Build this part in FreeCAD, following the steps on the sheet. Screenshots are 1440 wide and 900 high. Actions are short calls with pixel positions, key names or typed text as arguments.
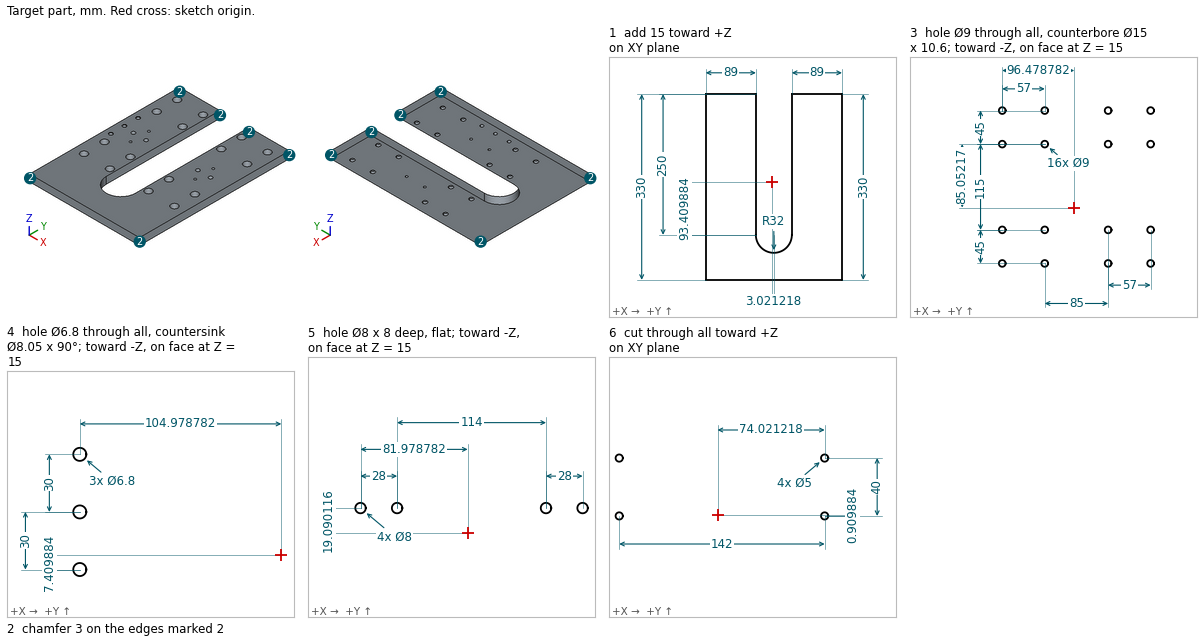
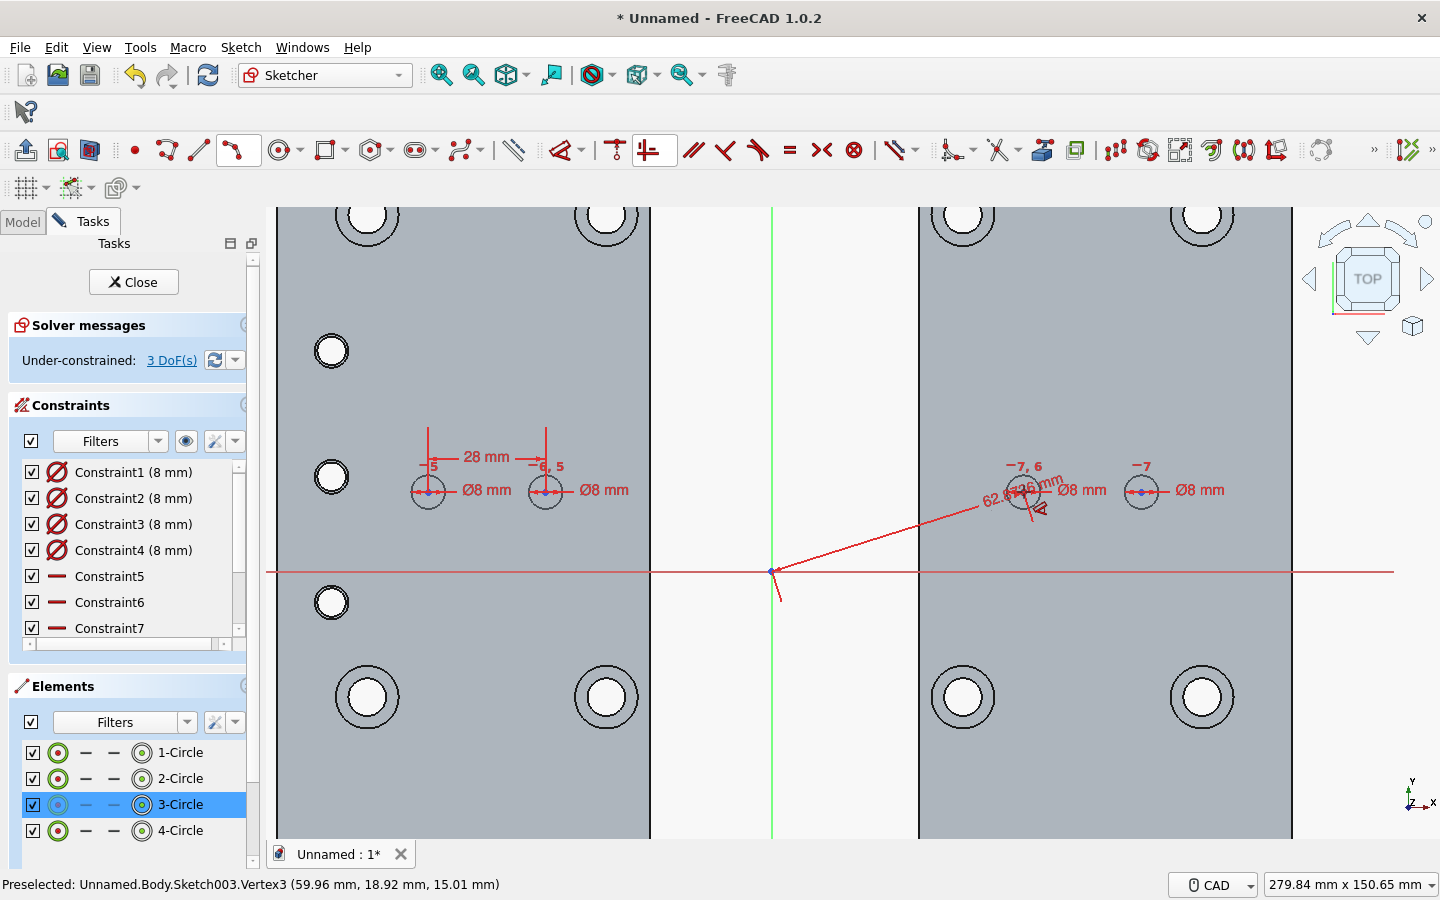
click(1142, 492)
click(1083, 458)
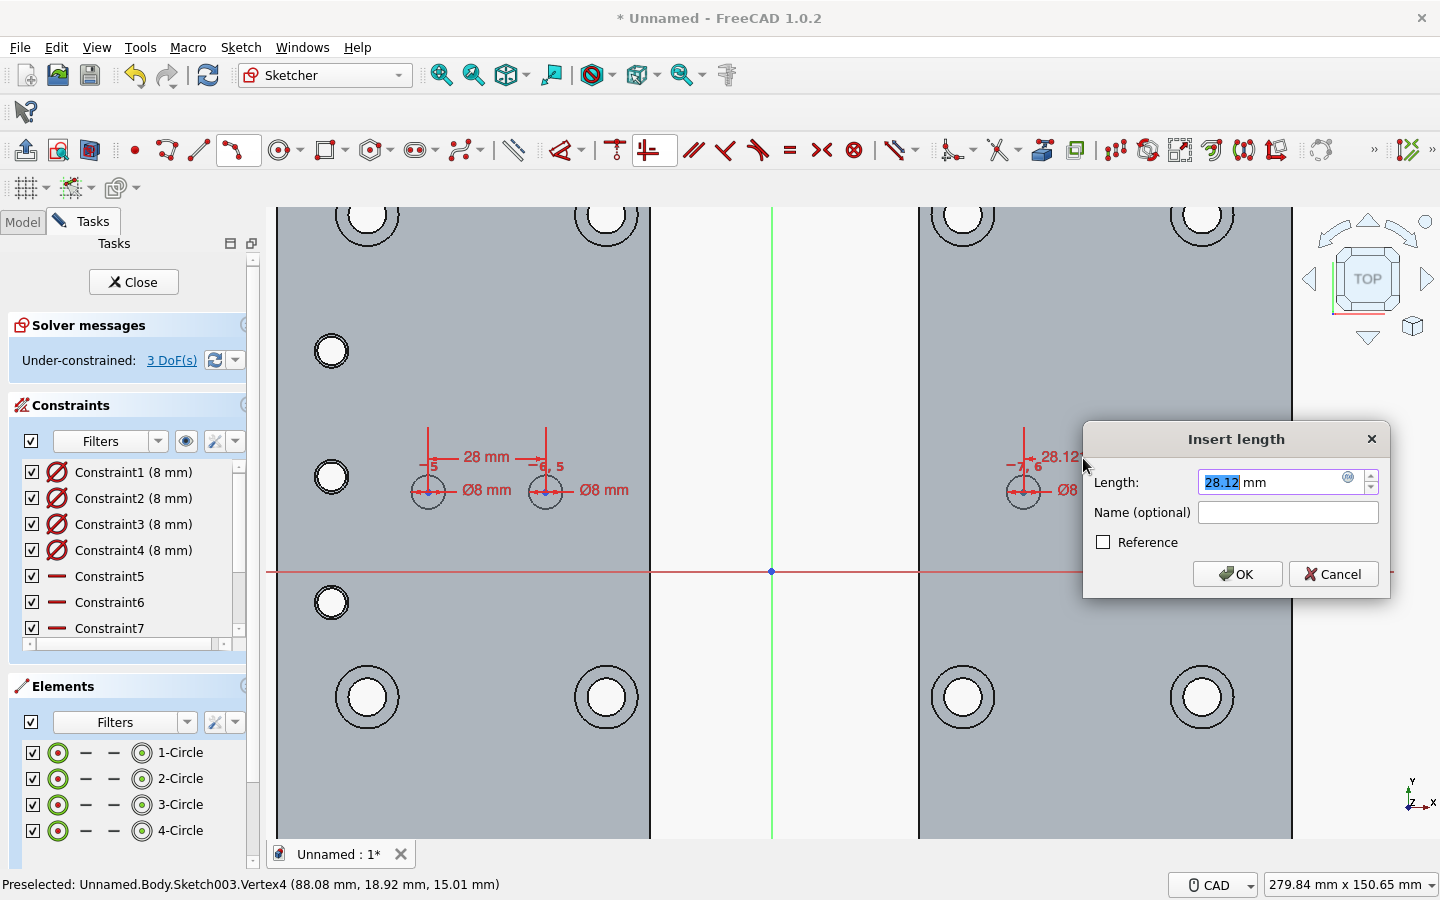
text(28)
key(Return)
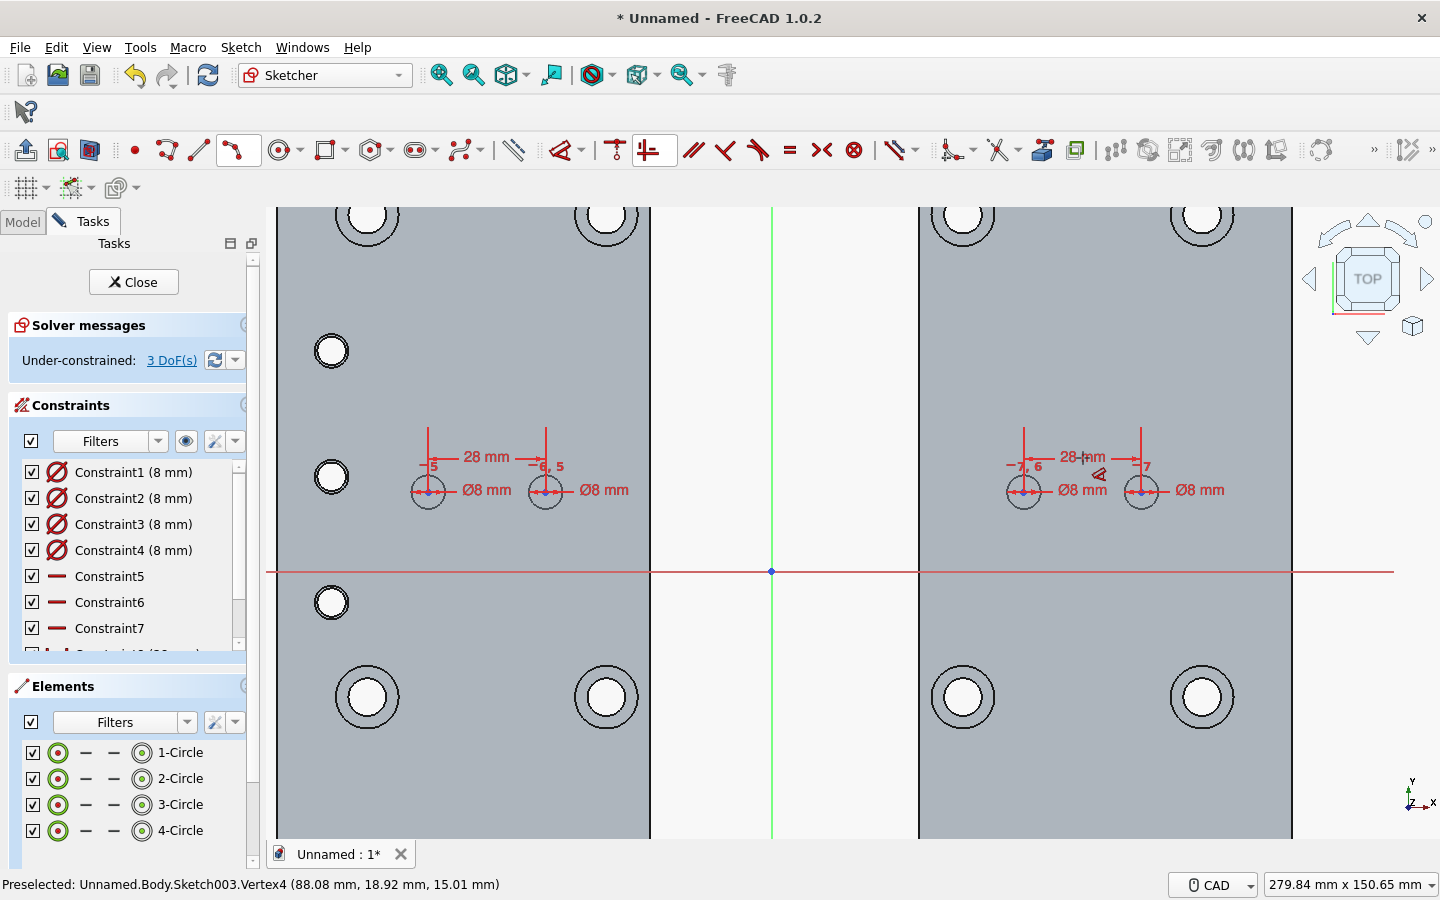
click(546, 492)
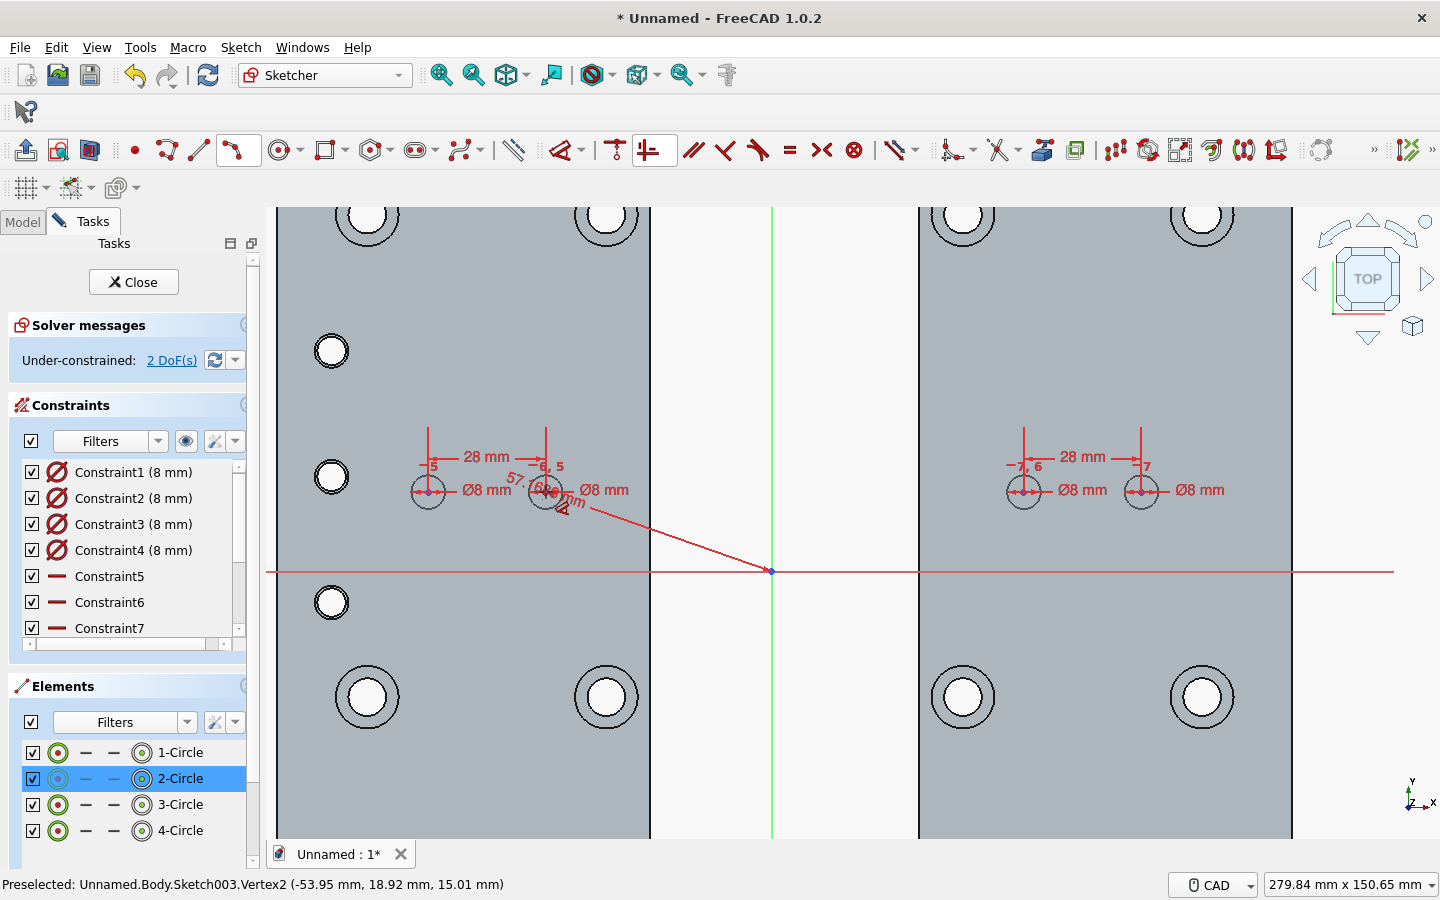
click(1024, 492)
click(675, 458)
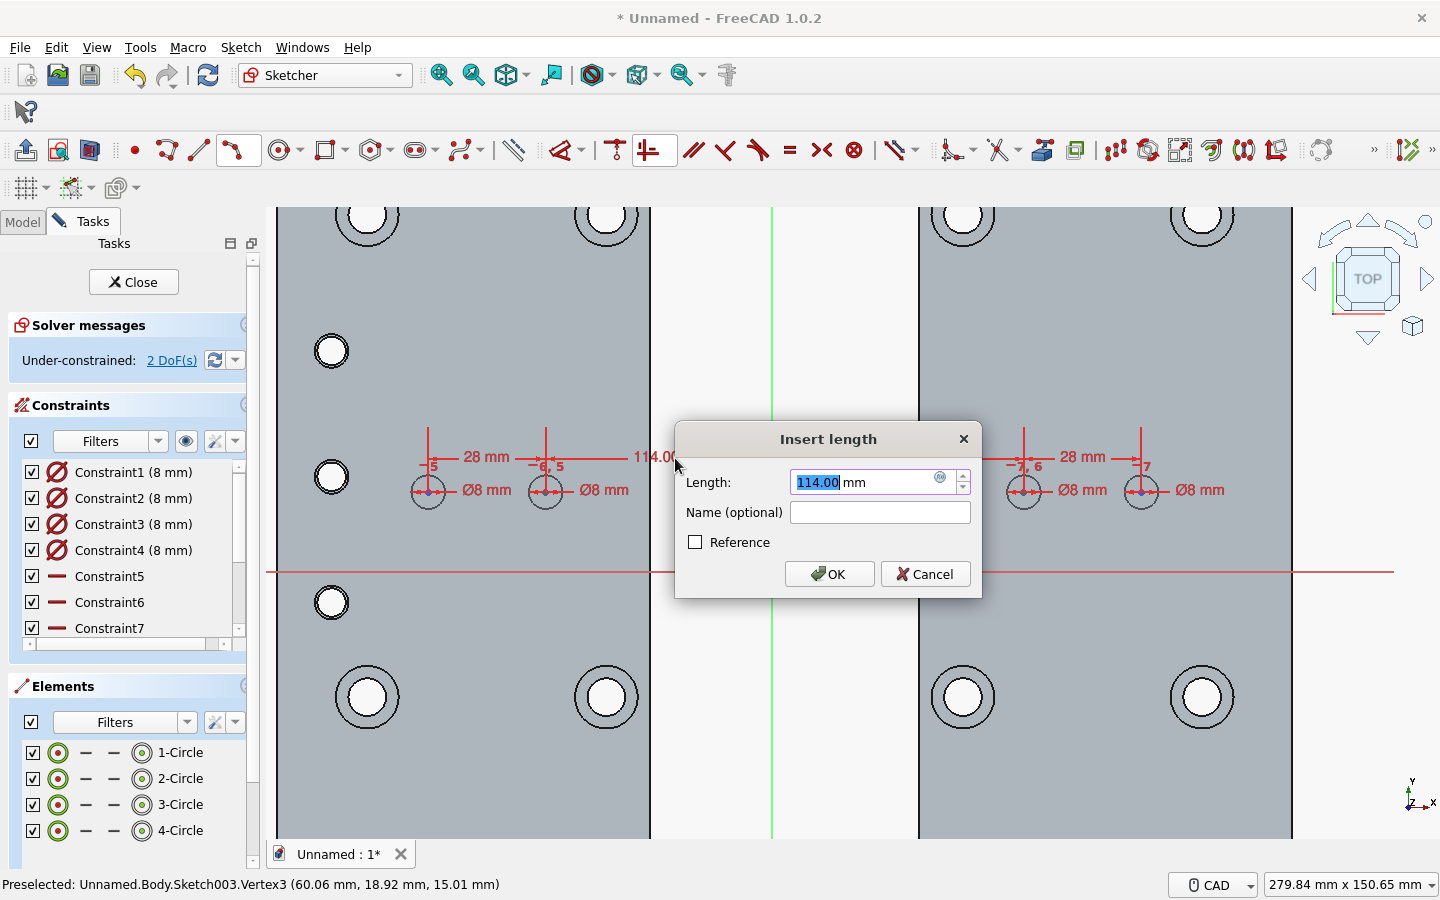
text(114)
key(Return)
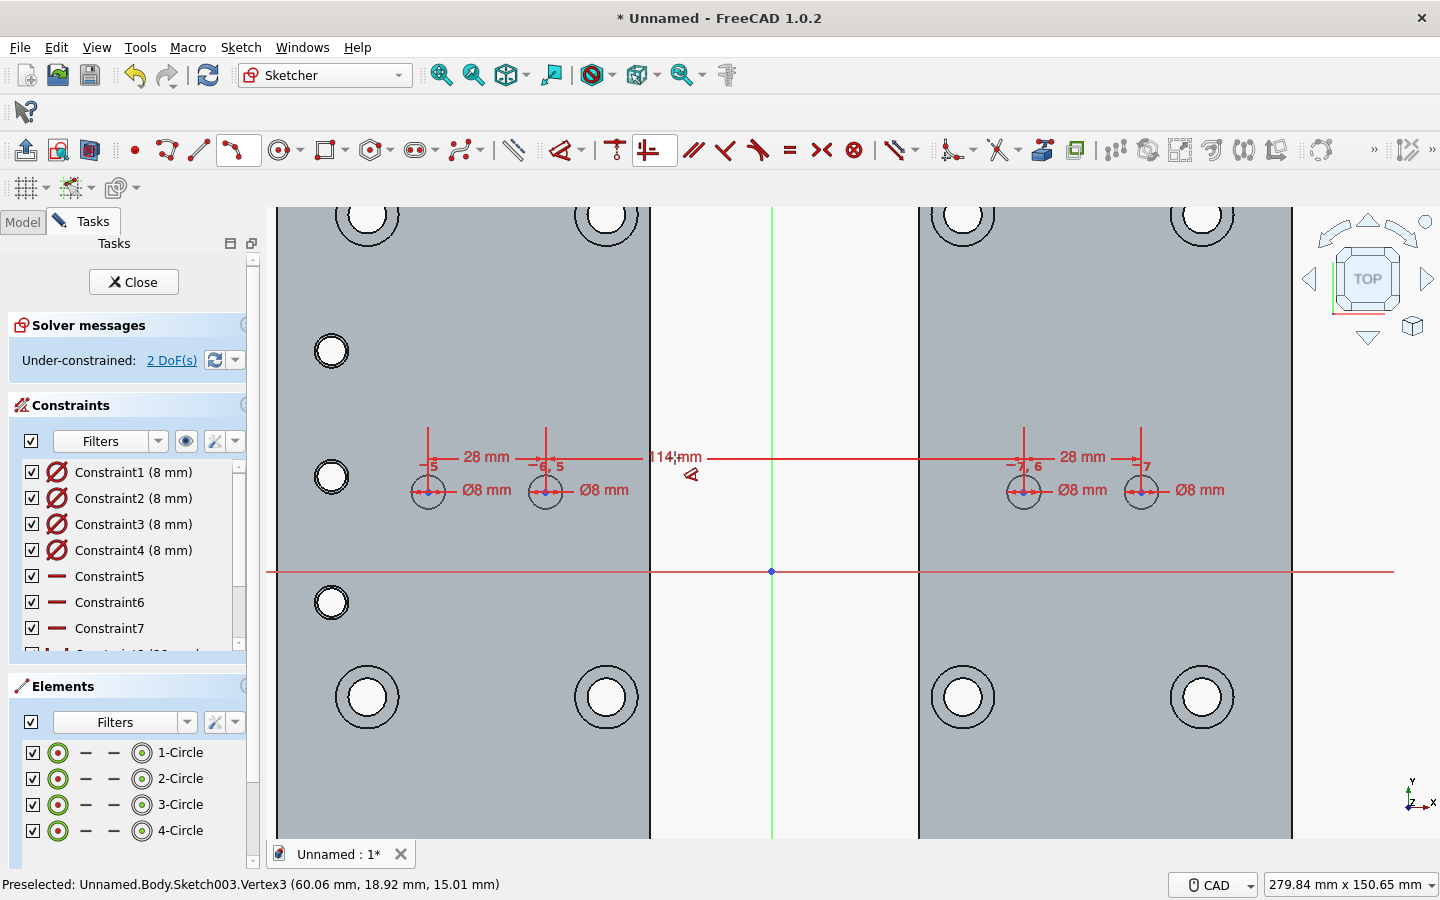
click(428, 492)
click(600, 606)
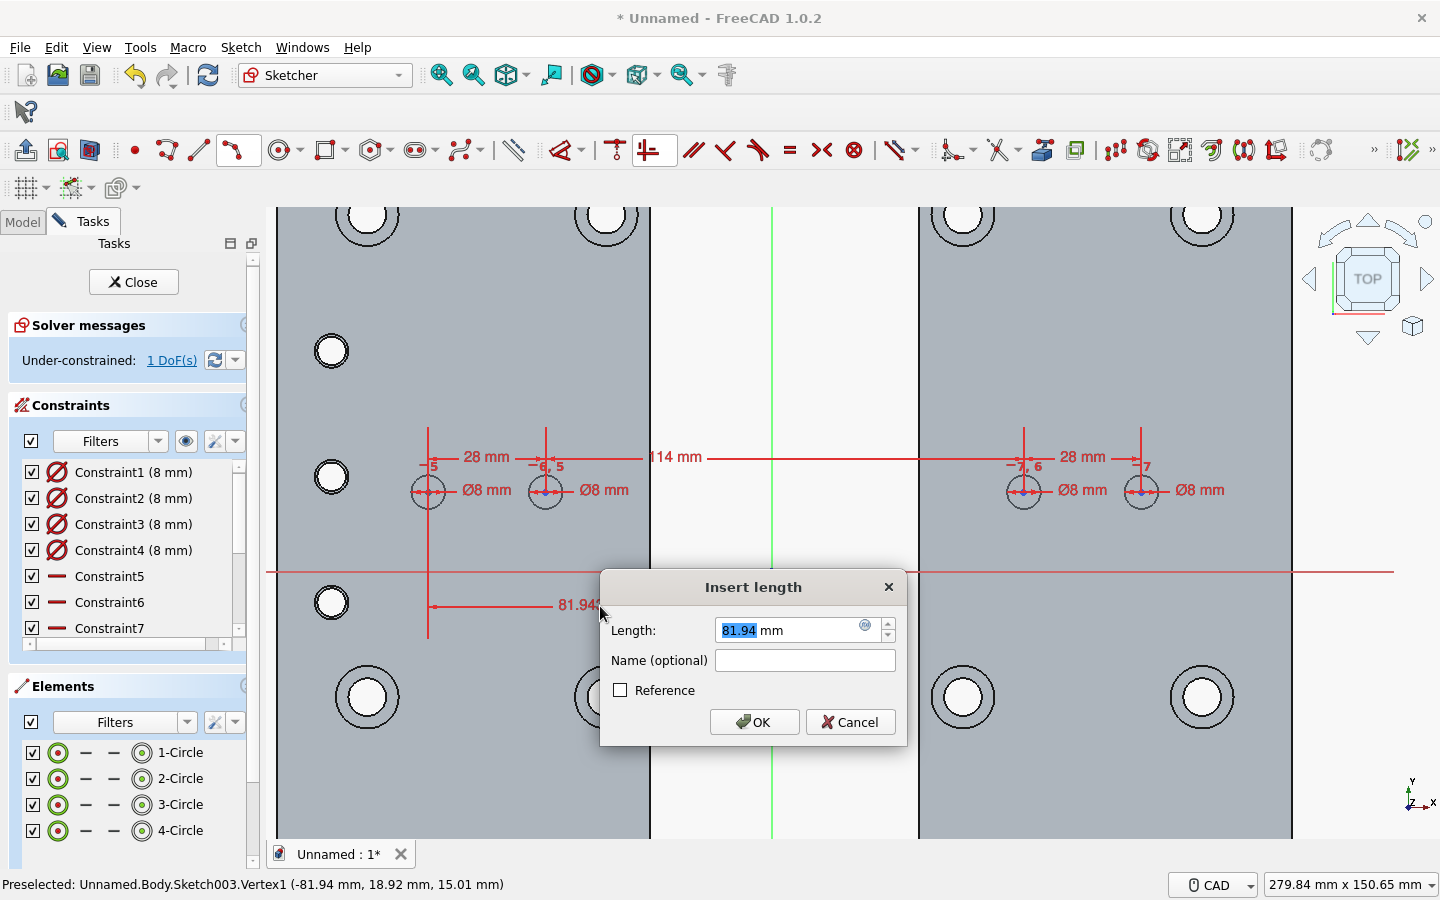
text(81.978782)
key(Return)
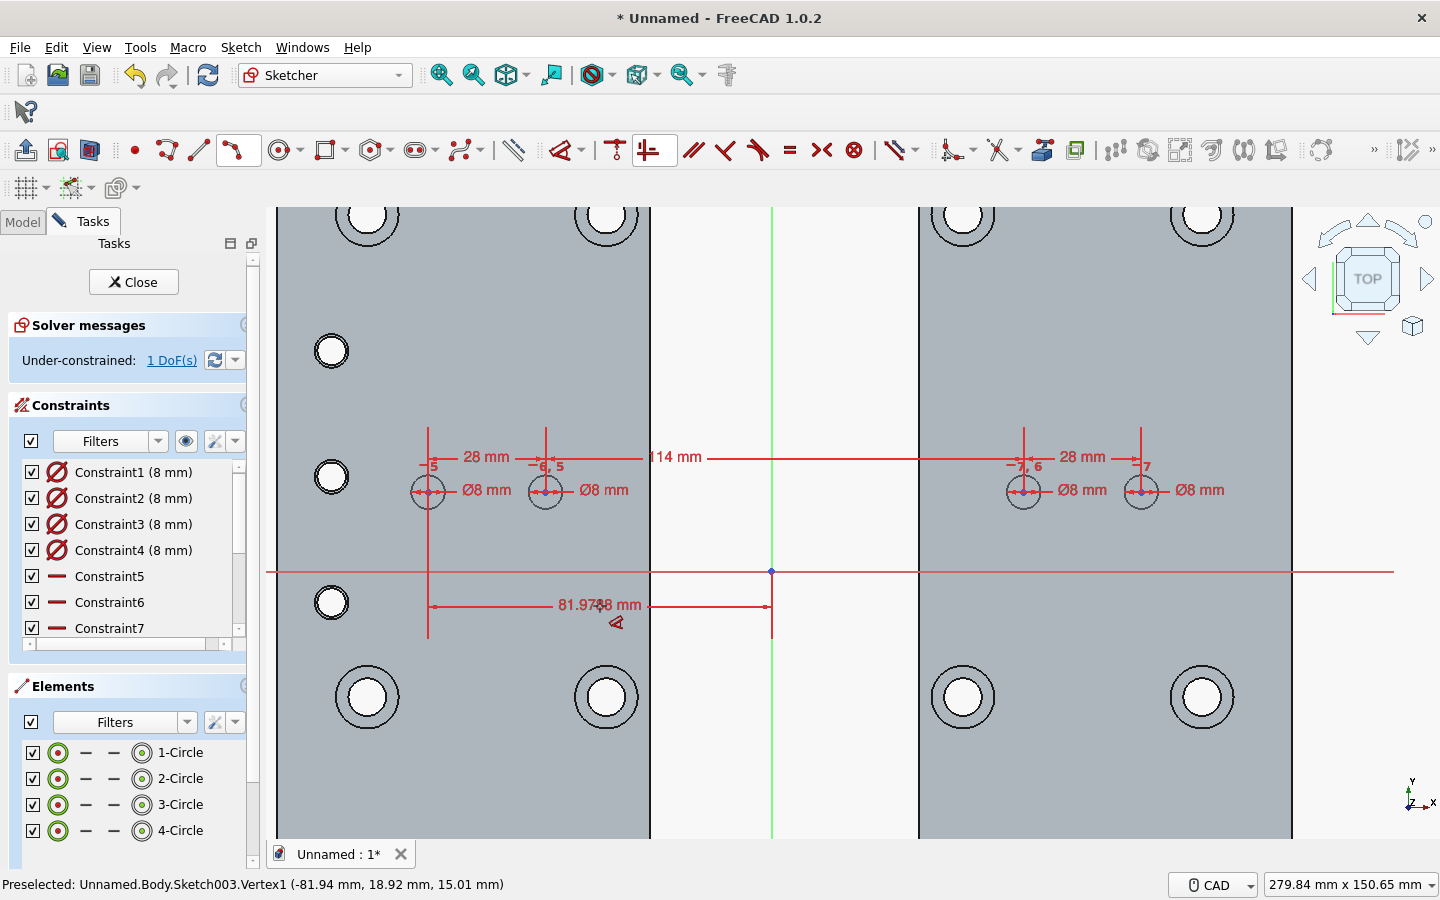
click(428, 492)
click(394, 532)